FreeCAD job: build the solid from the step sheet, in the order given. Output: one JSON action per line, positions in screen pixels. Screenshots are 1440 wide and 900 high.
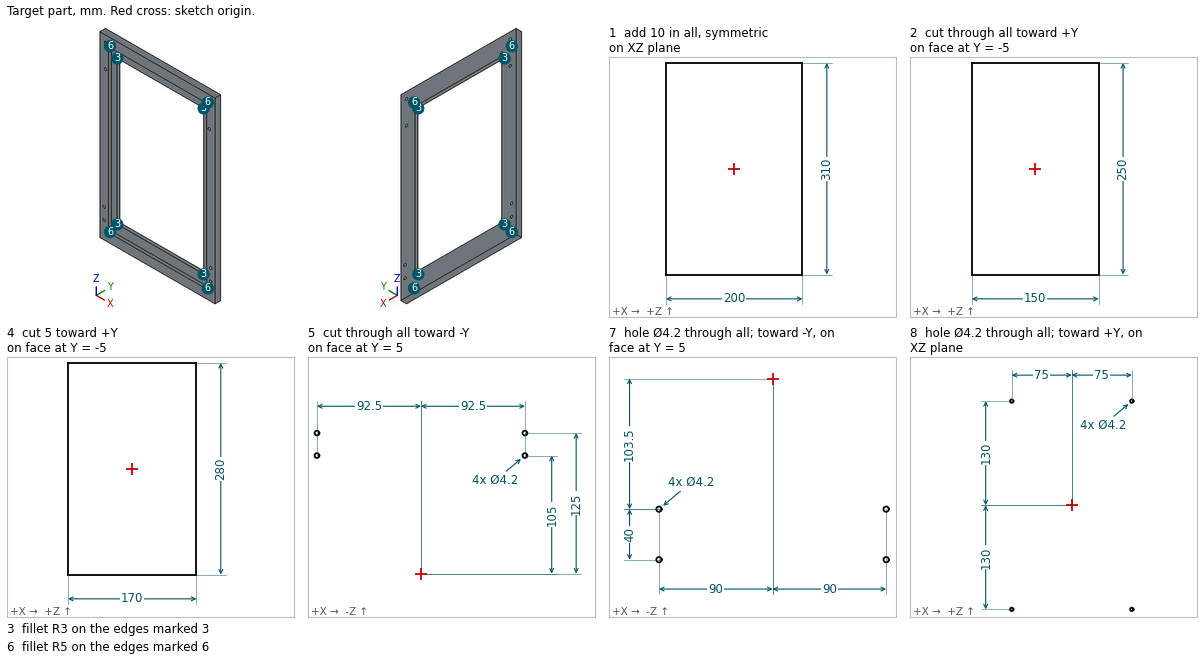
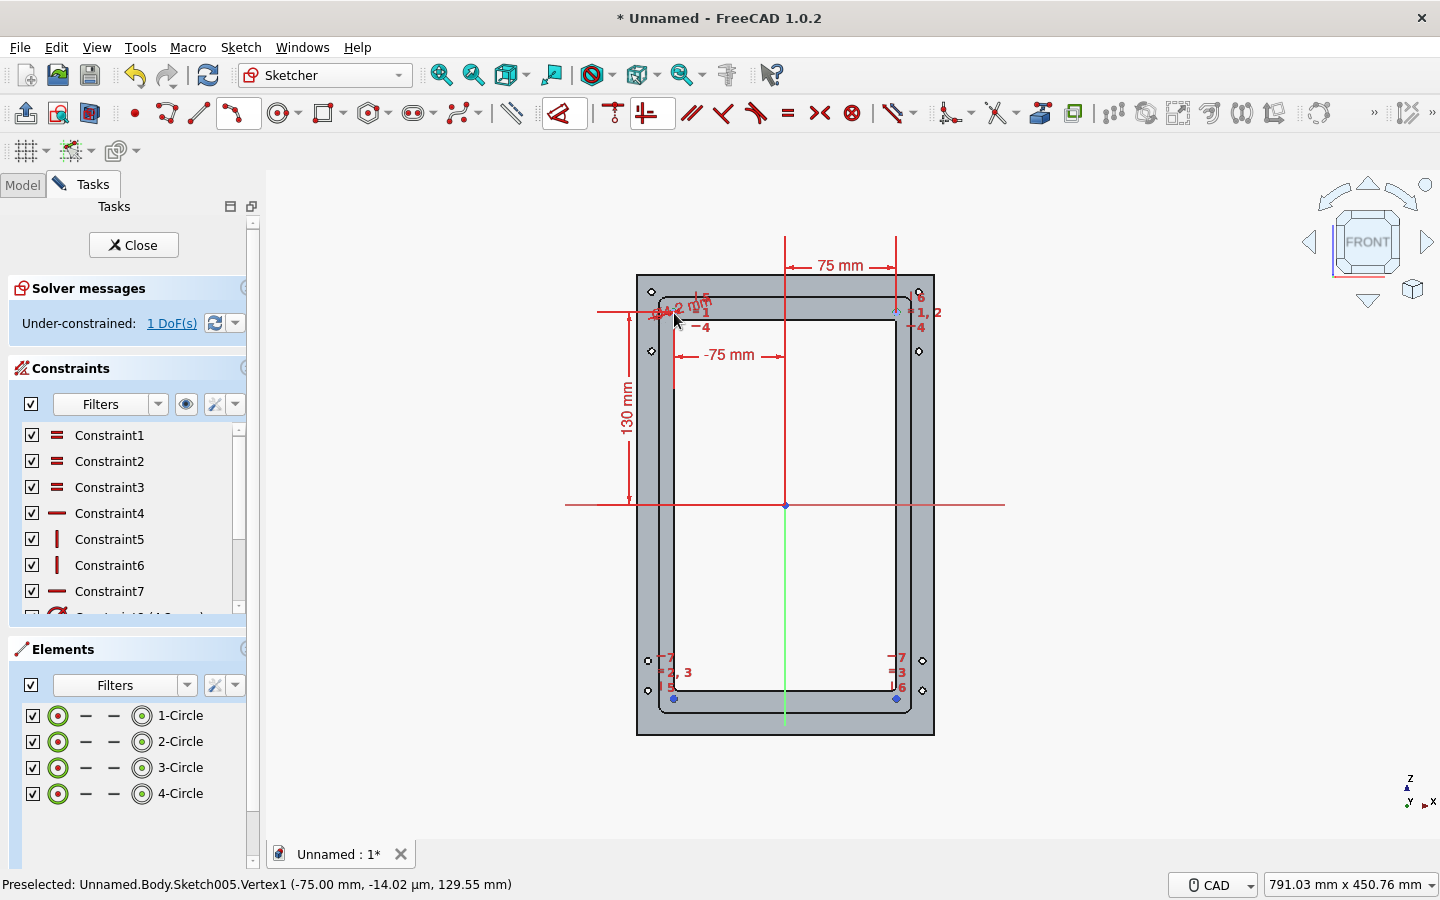
{"action": "left_click", "coordinate": [674, 699]}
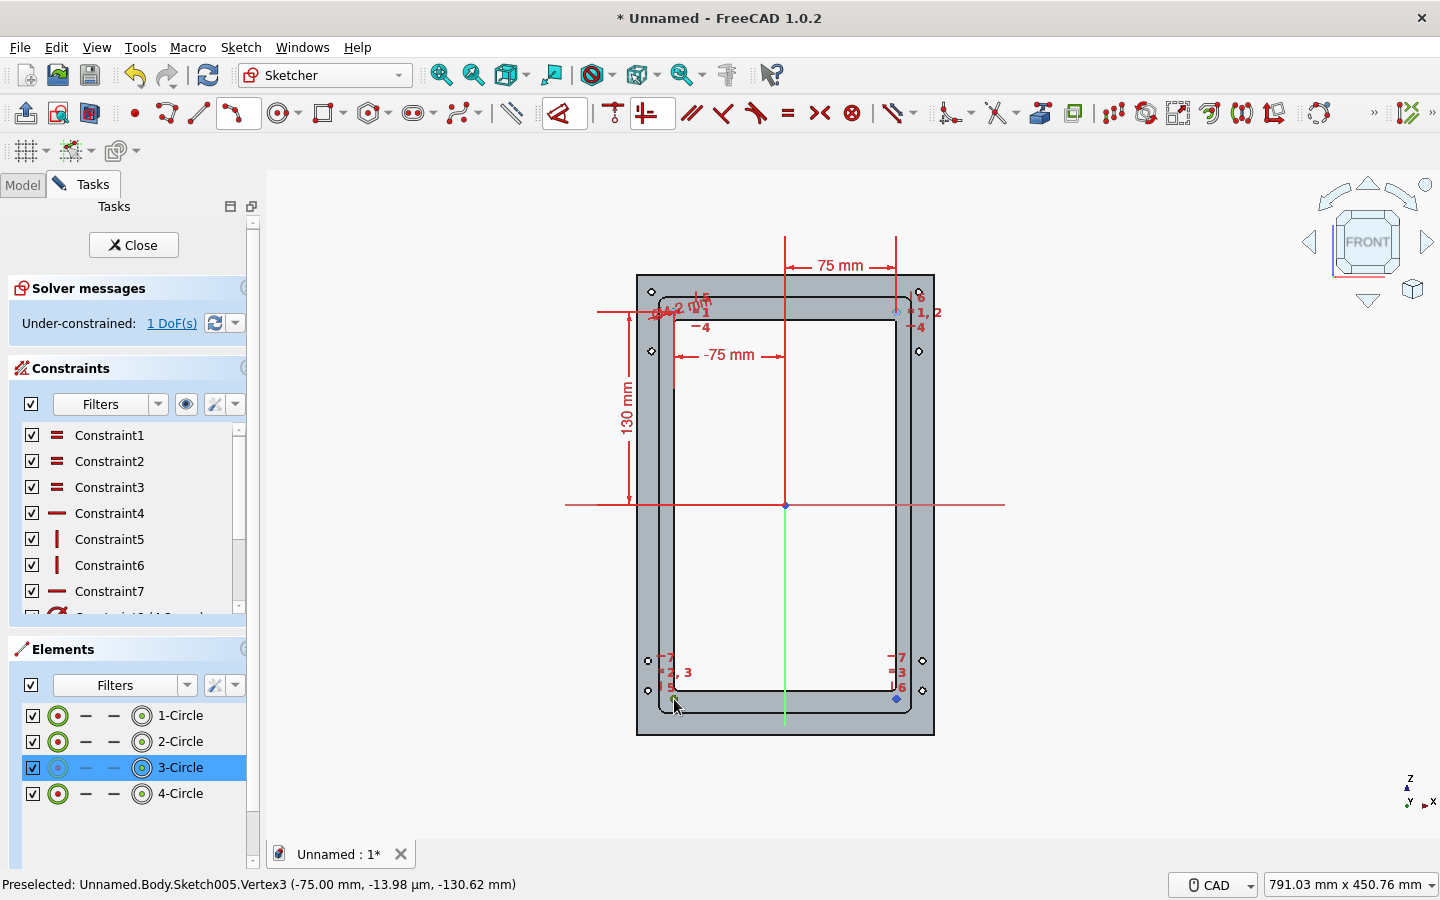
{"action": "key", "text": "i"}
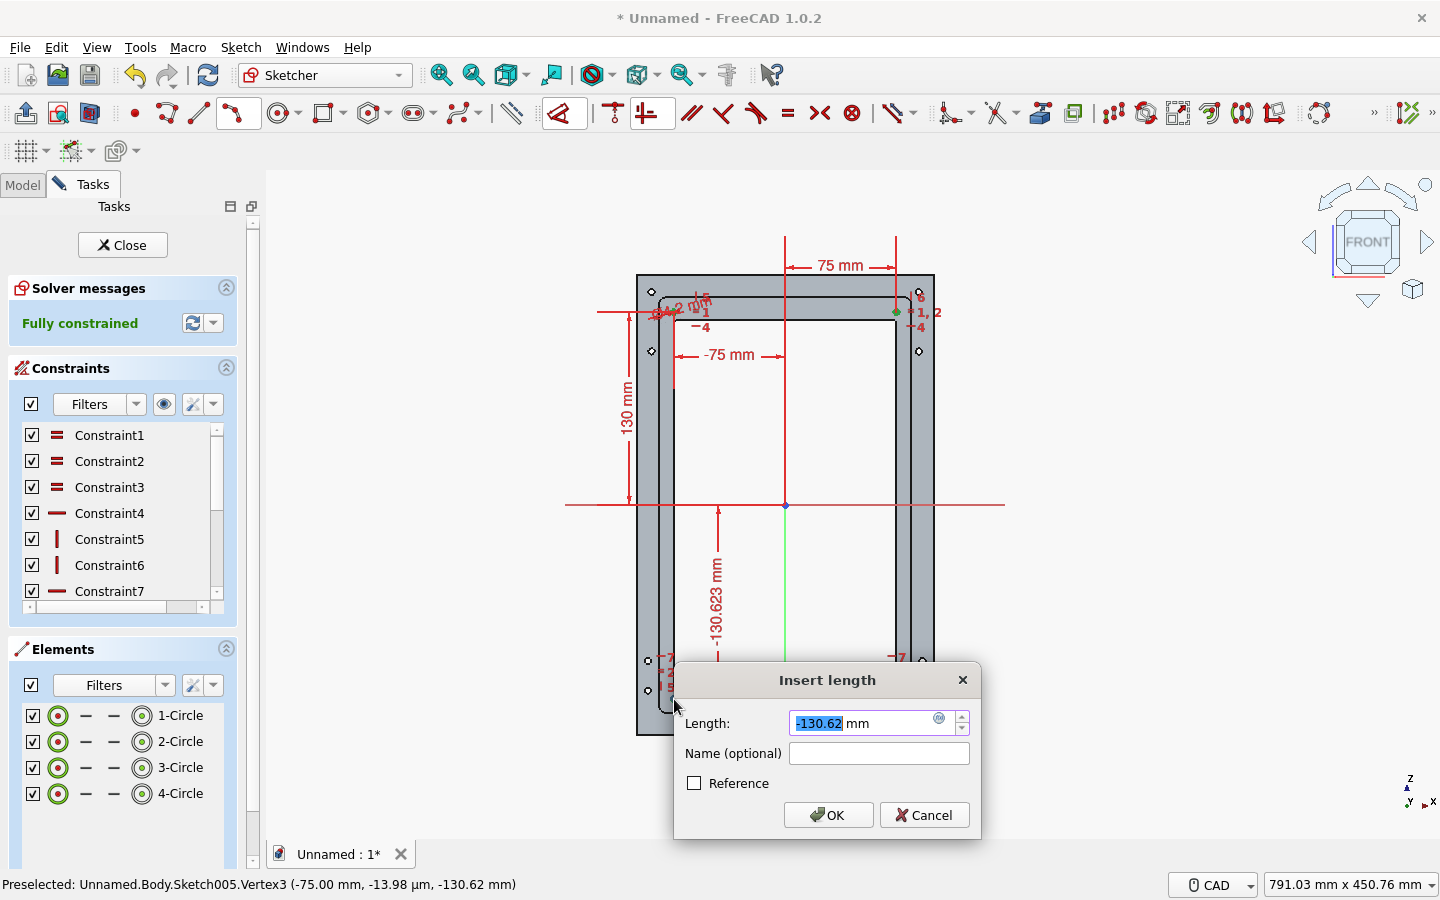
{"action": "type", "text": "-130"}
{"action": "key", "text": "Return"}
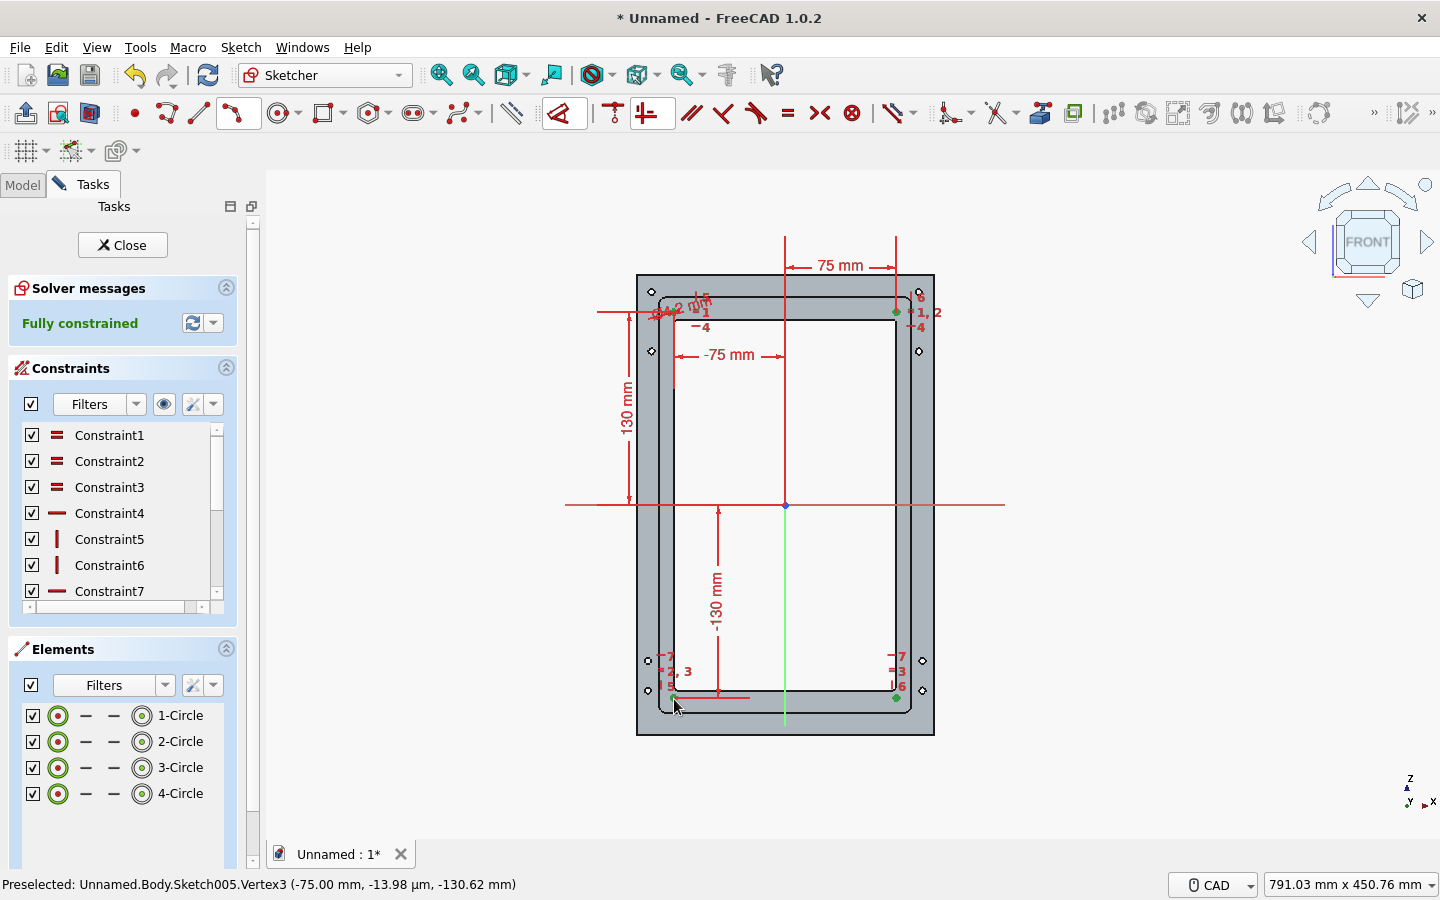
{"action": "left_click", "coordinate": [123, 245]}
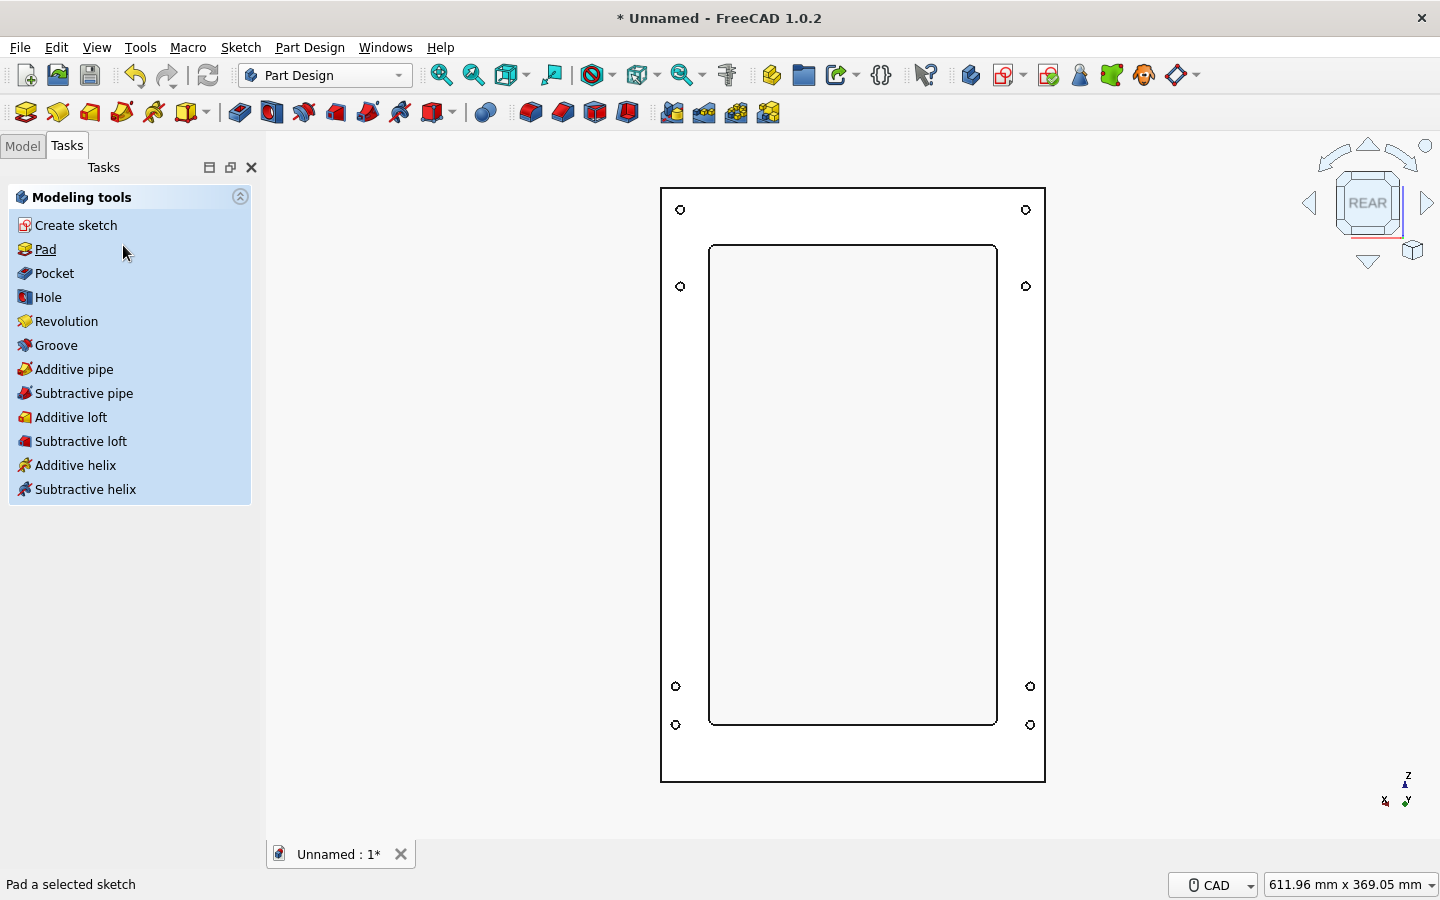
{"action": "left_click", "coordinate": [272, 112]}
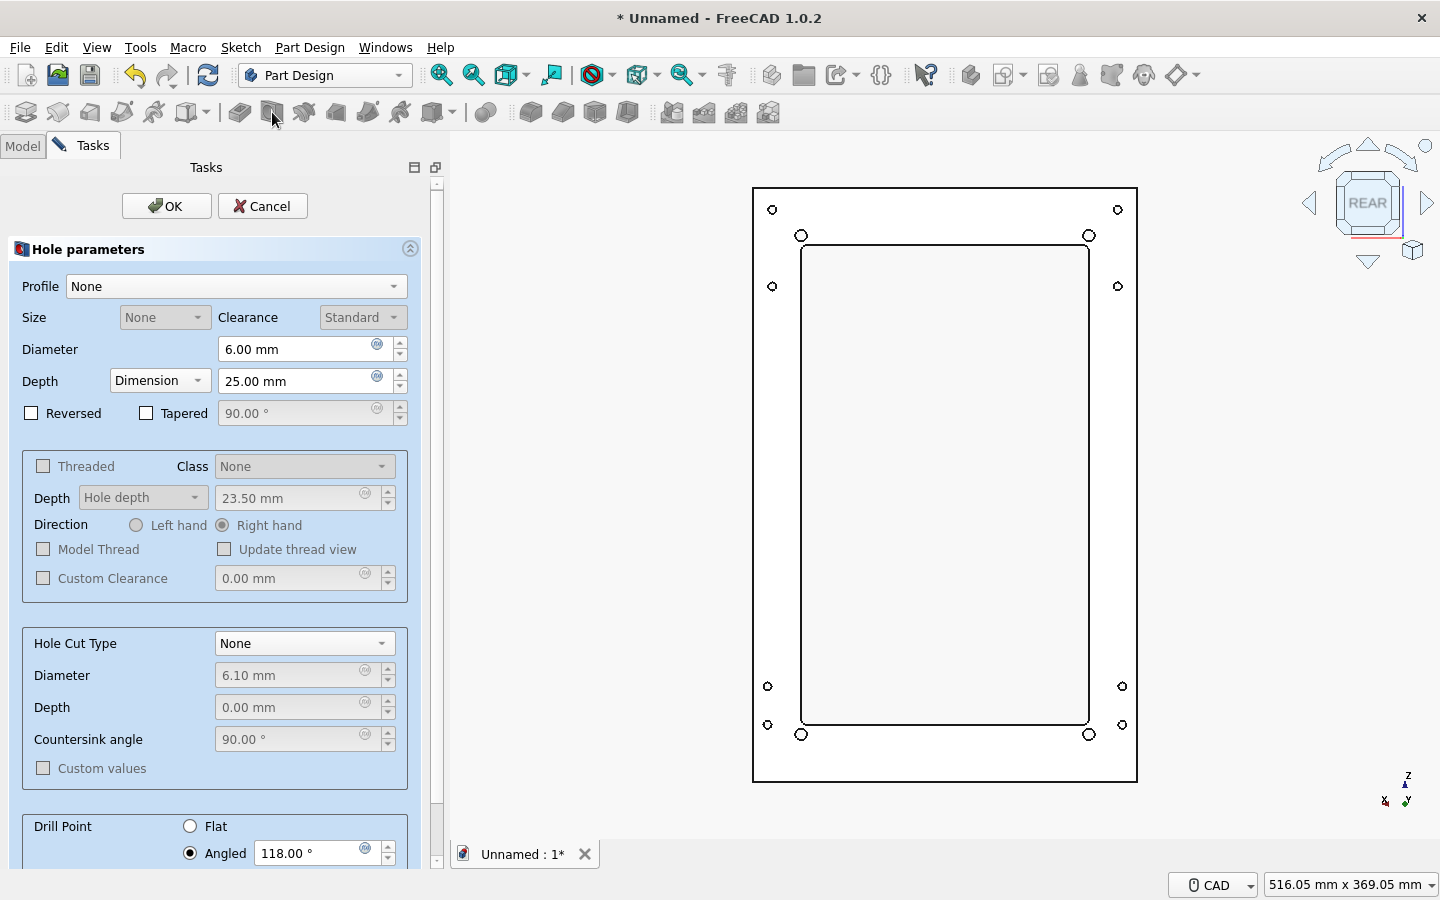
{"action": "triple_click", "coordinate": [305, 349]}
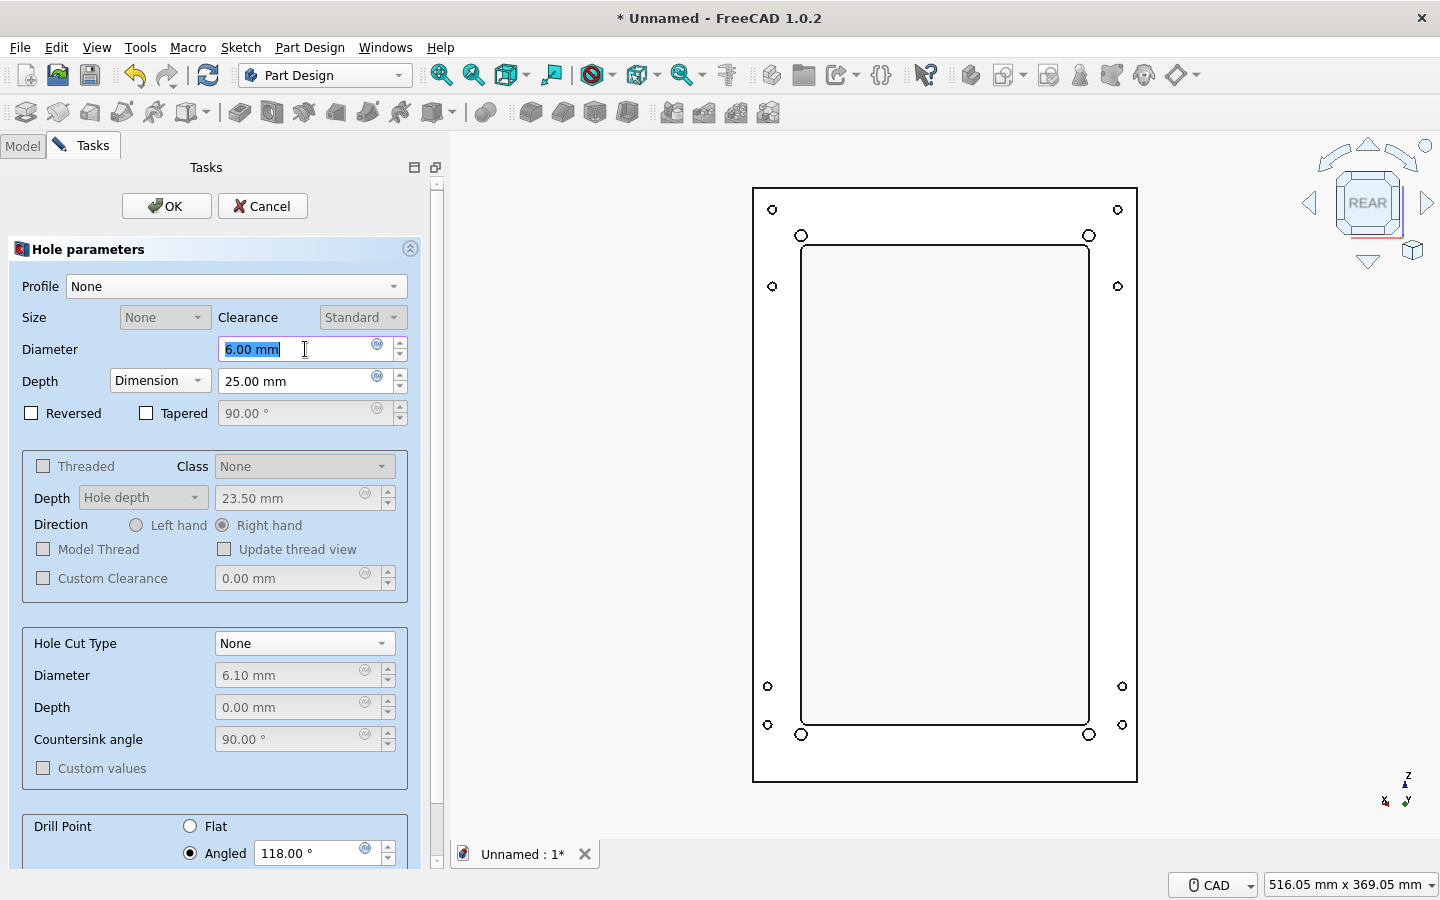
{"action": "type", "text": "4.2"}
{"action": "key", "text": "Tab"}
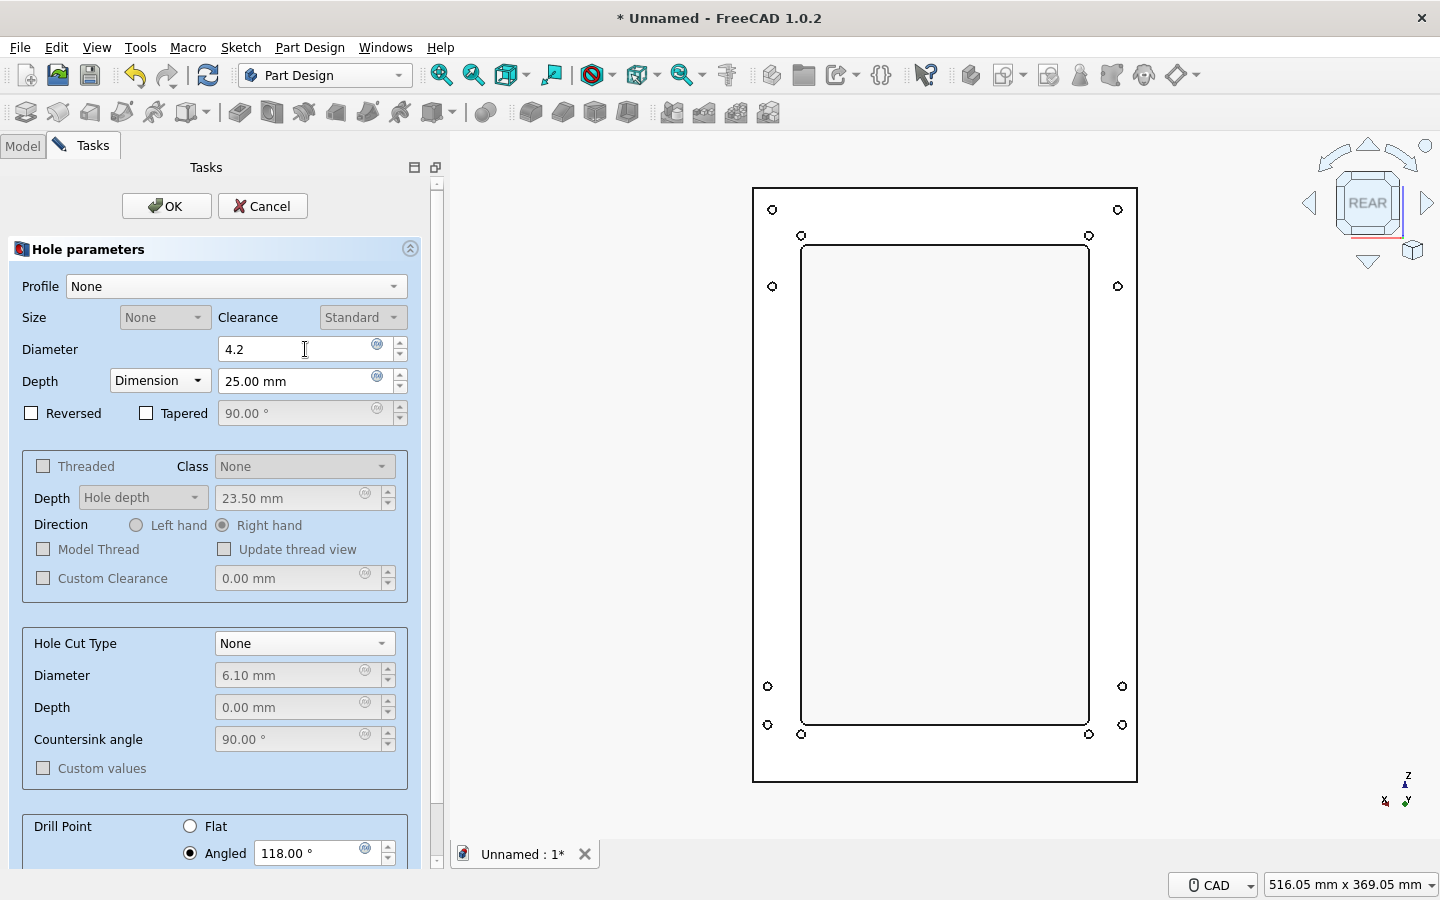
{"action": "left_click", "coordinate": [161, 380]}